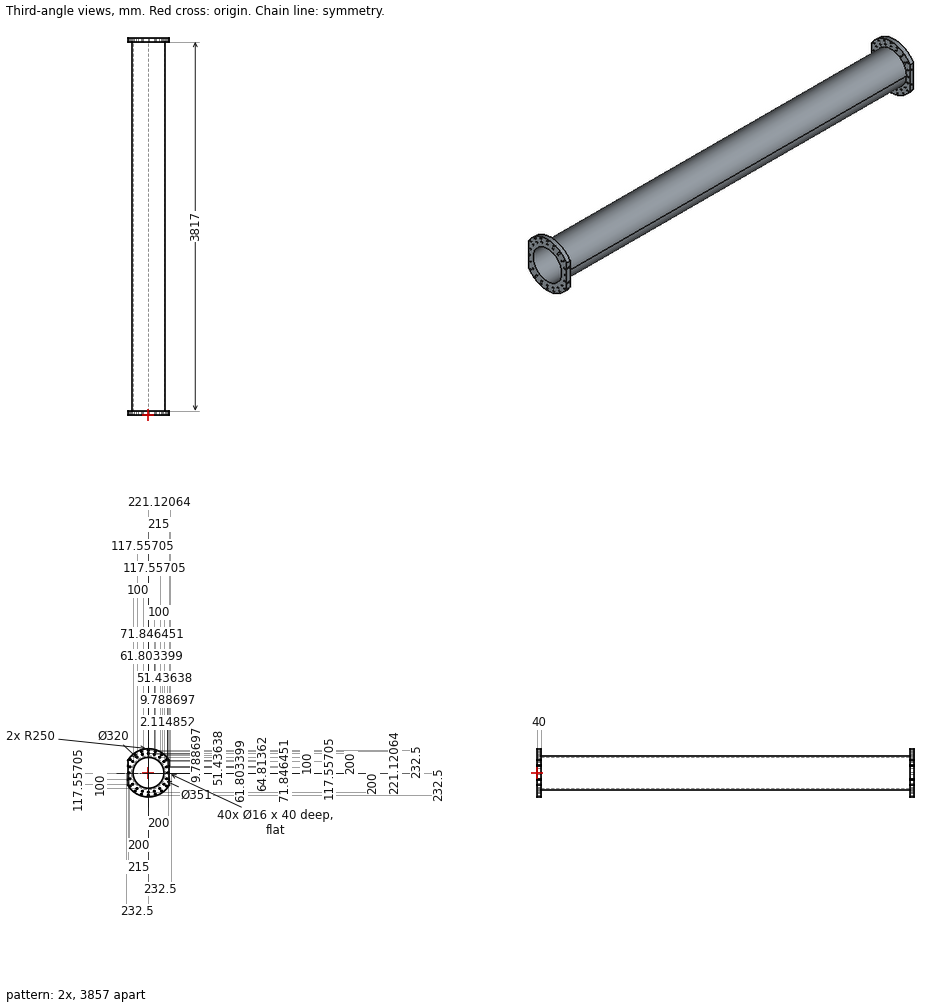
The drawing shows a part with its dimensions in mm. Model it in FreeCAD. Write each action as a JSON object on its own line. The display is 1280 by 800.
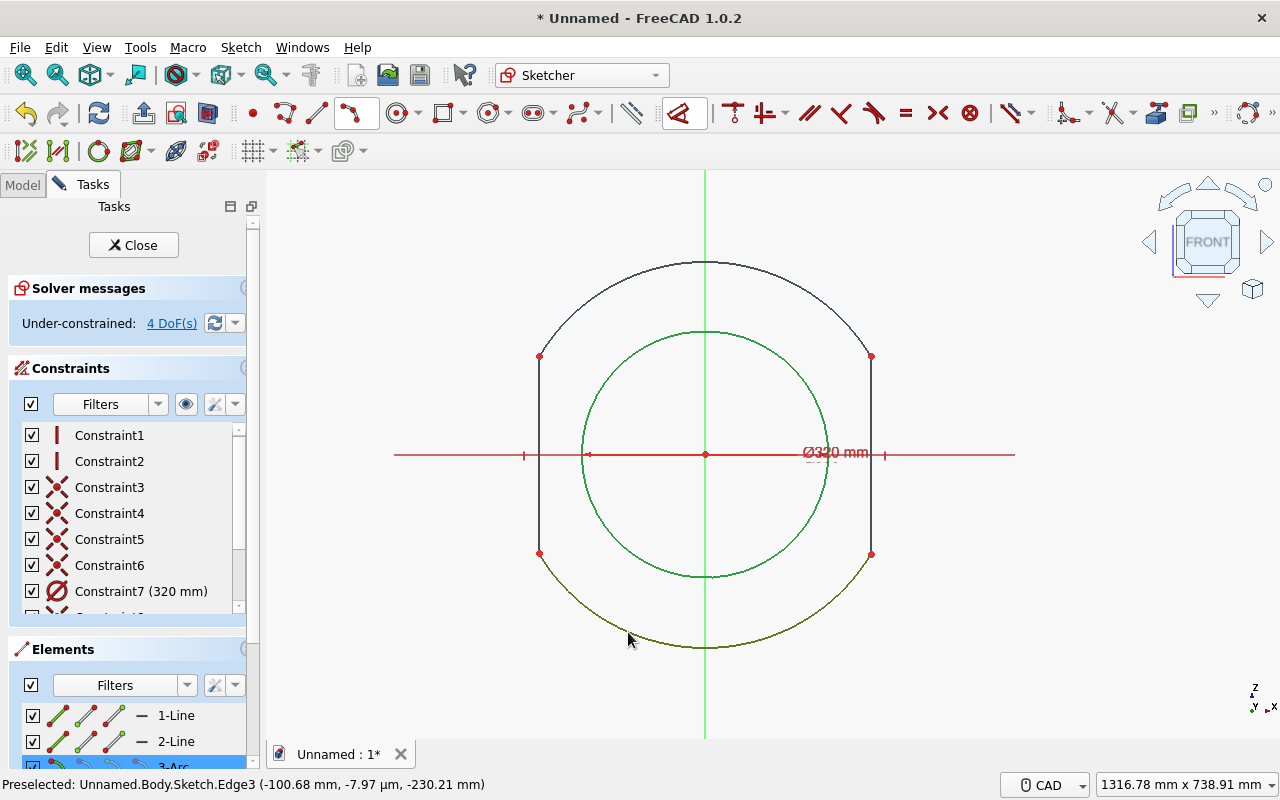
{"action": "left_click", "coordinate": [783, 278]}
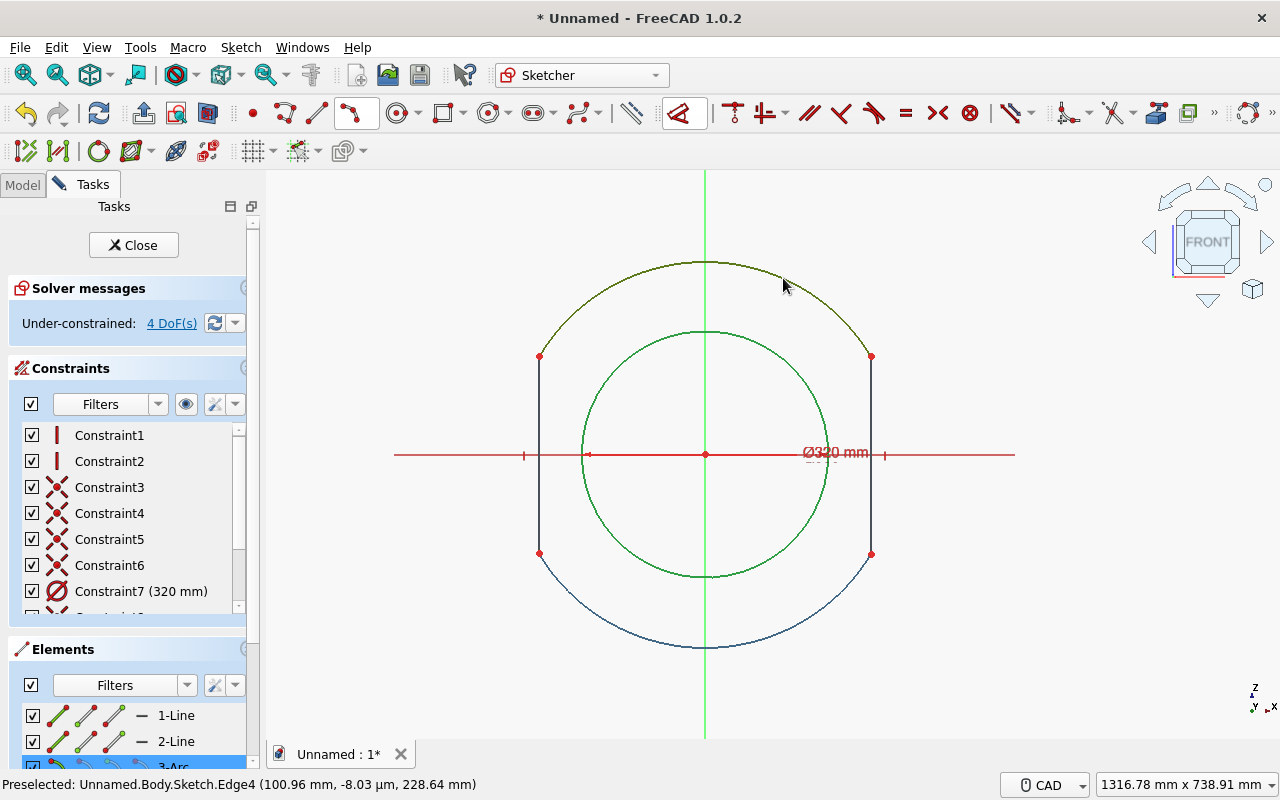
{"action": "left_click", "coordinate": [906, 114]}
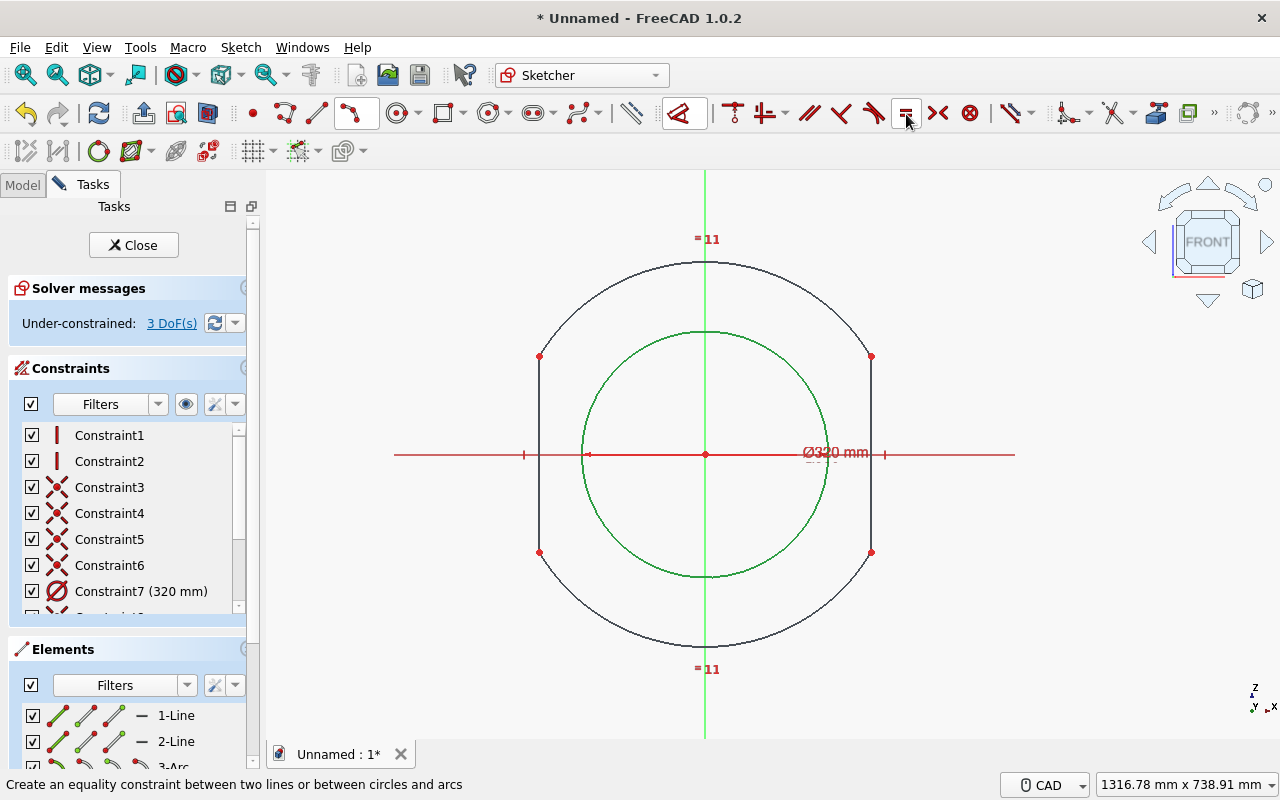
{"action": "left_click", "coordinate": [627, 631]}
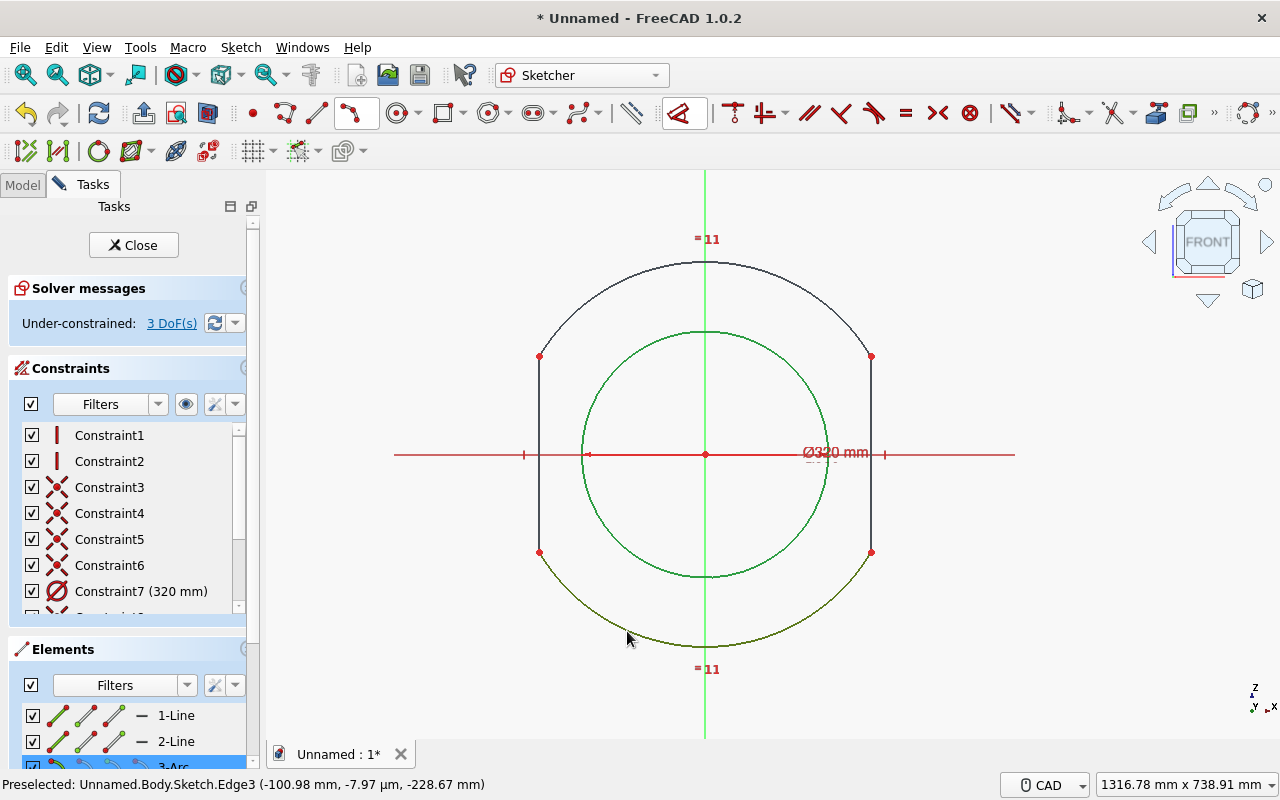
{"action": "left_click", "coordinate": [702, 114]}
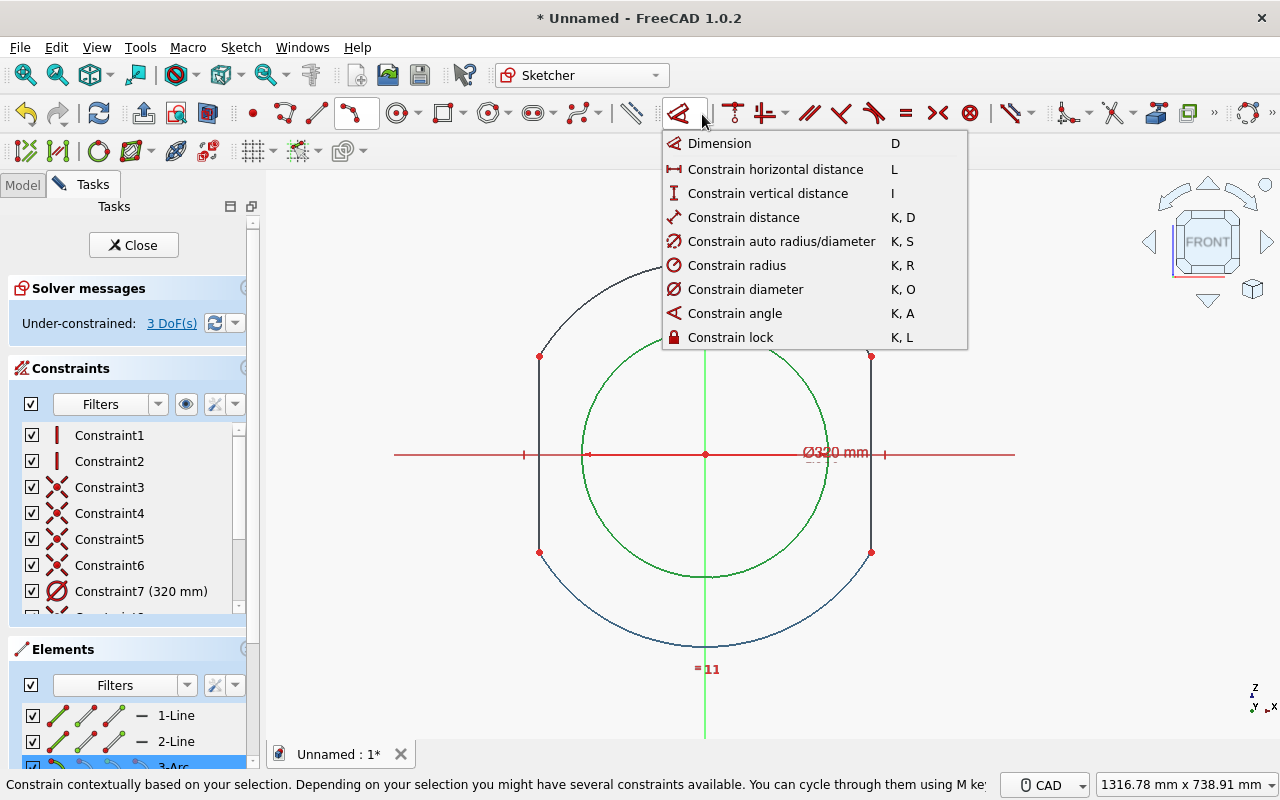
{"action": "left_click", "coordinate": [815, 265]}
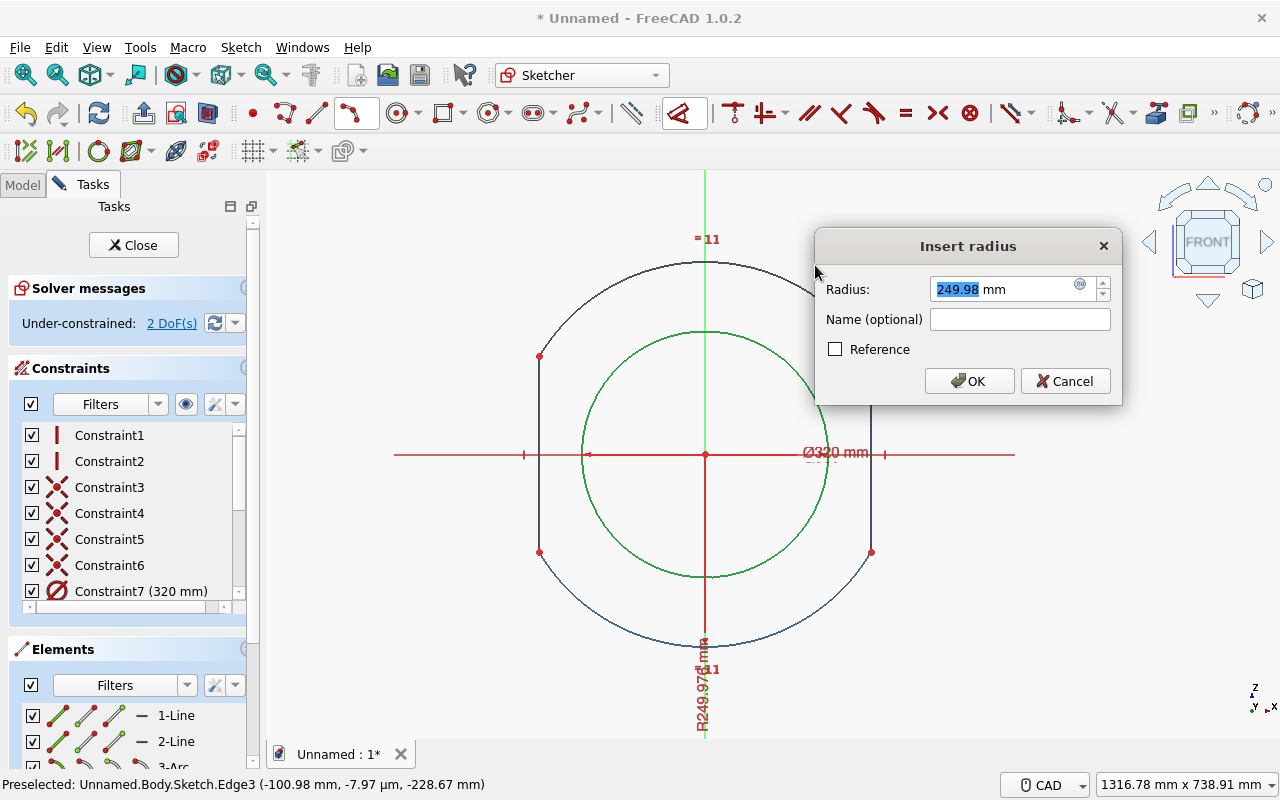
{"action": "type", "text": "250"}
{"action": "key", "text": "Return"}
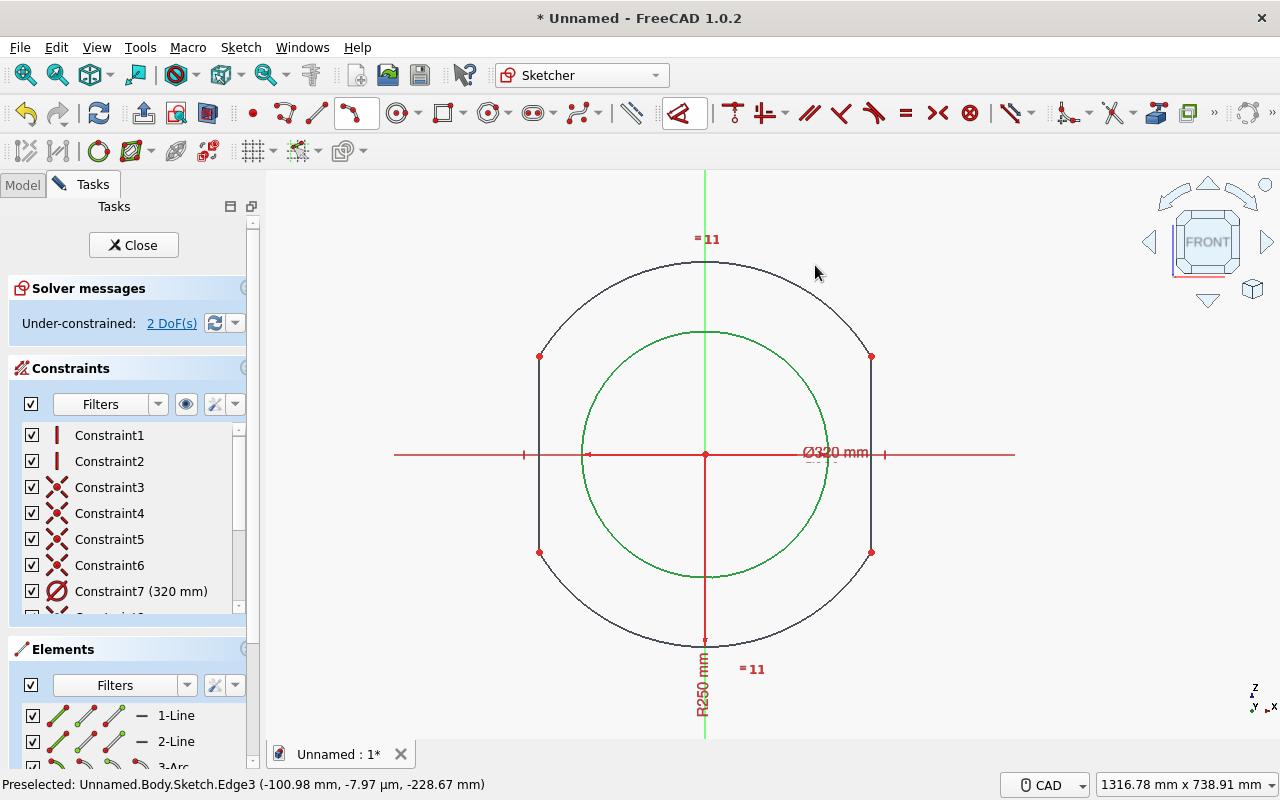
{"action": "left_click", "coordinate": [871, 357]}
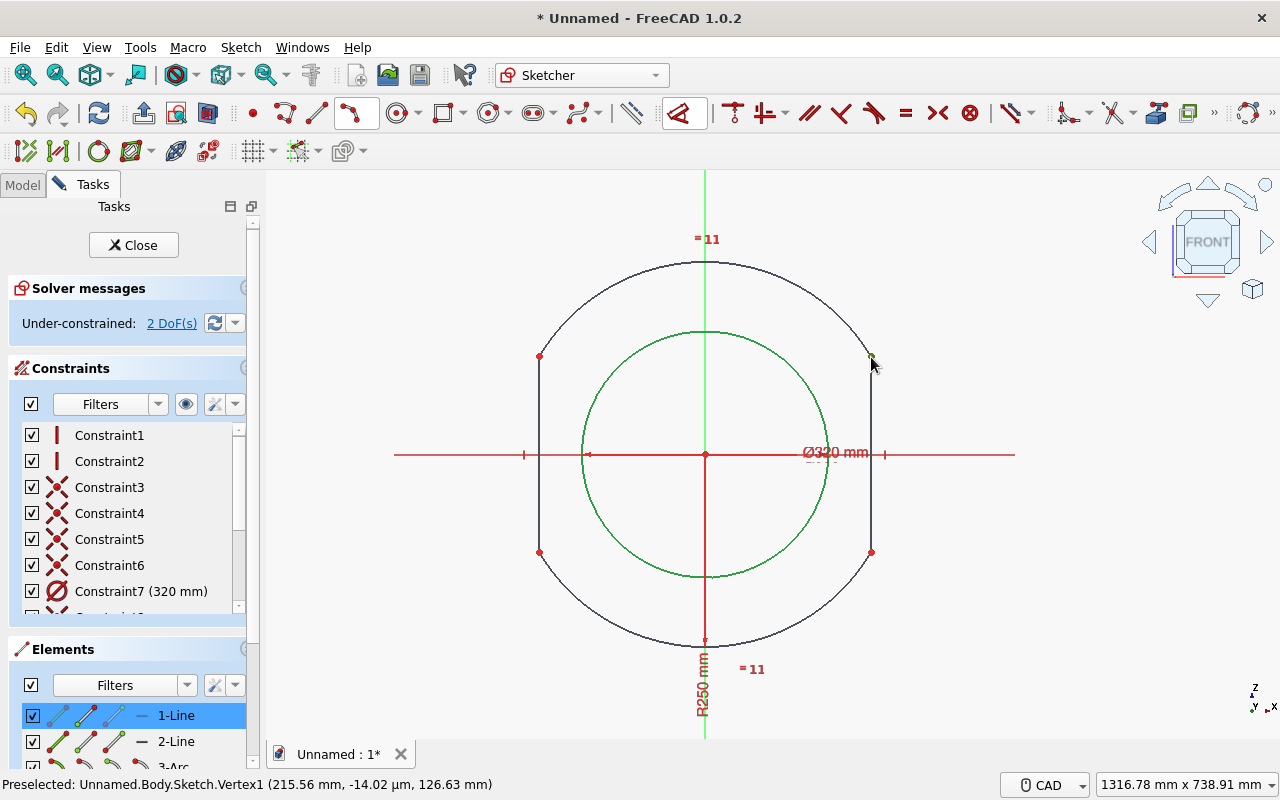
{"action": "left_click", "coordinate": [702, 114]}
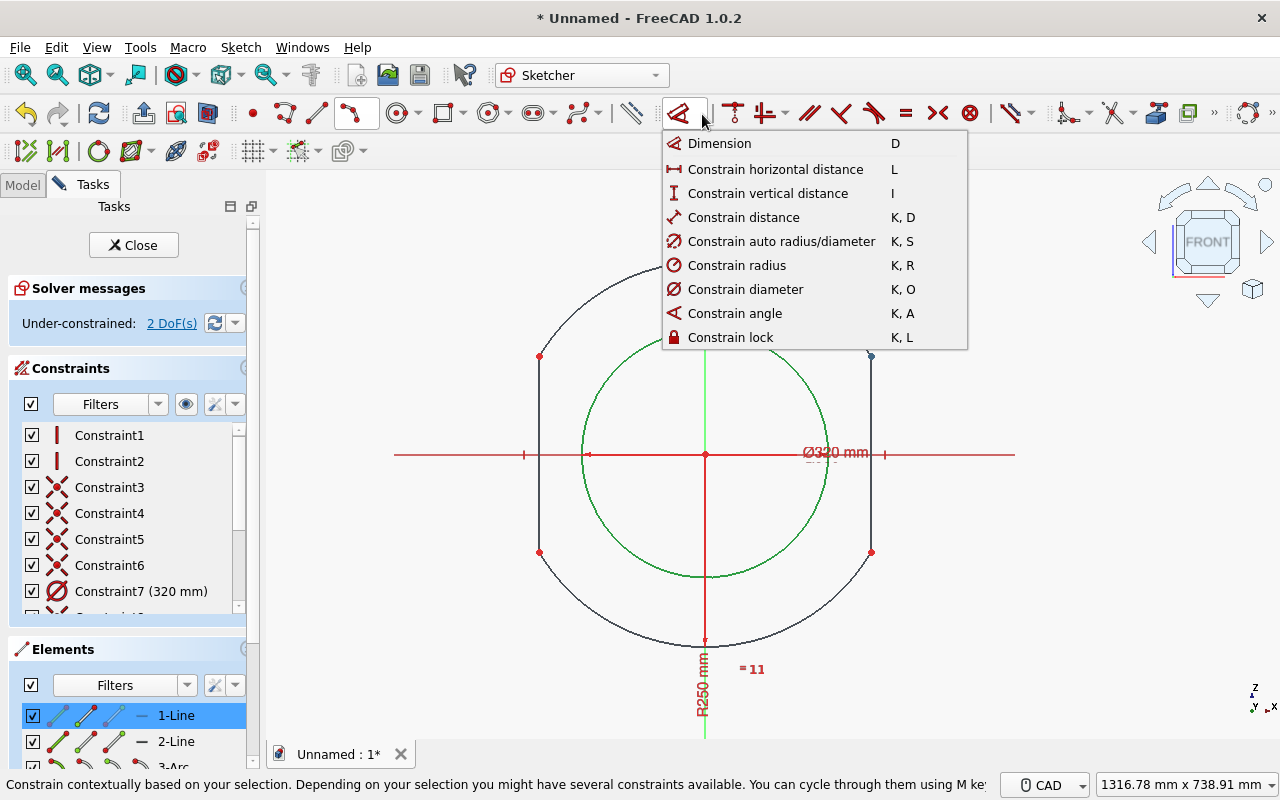
{"action": "left_click", "coordinate": [815, 169]}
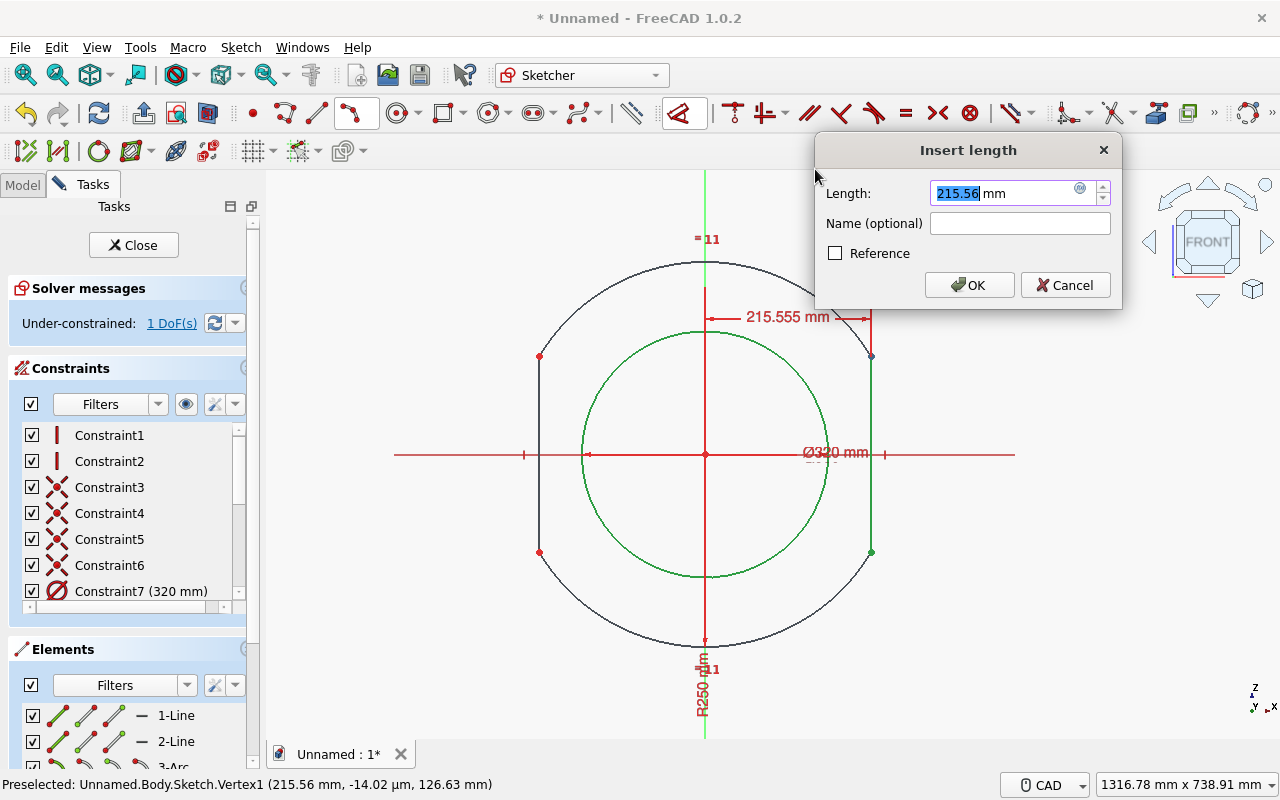
{"action": "type", "text": "215"}
{"action": "key", "text": "Return"}